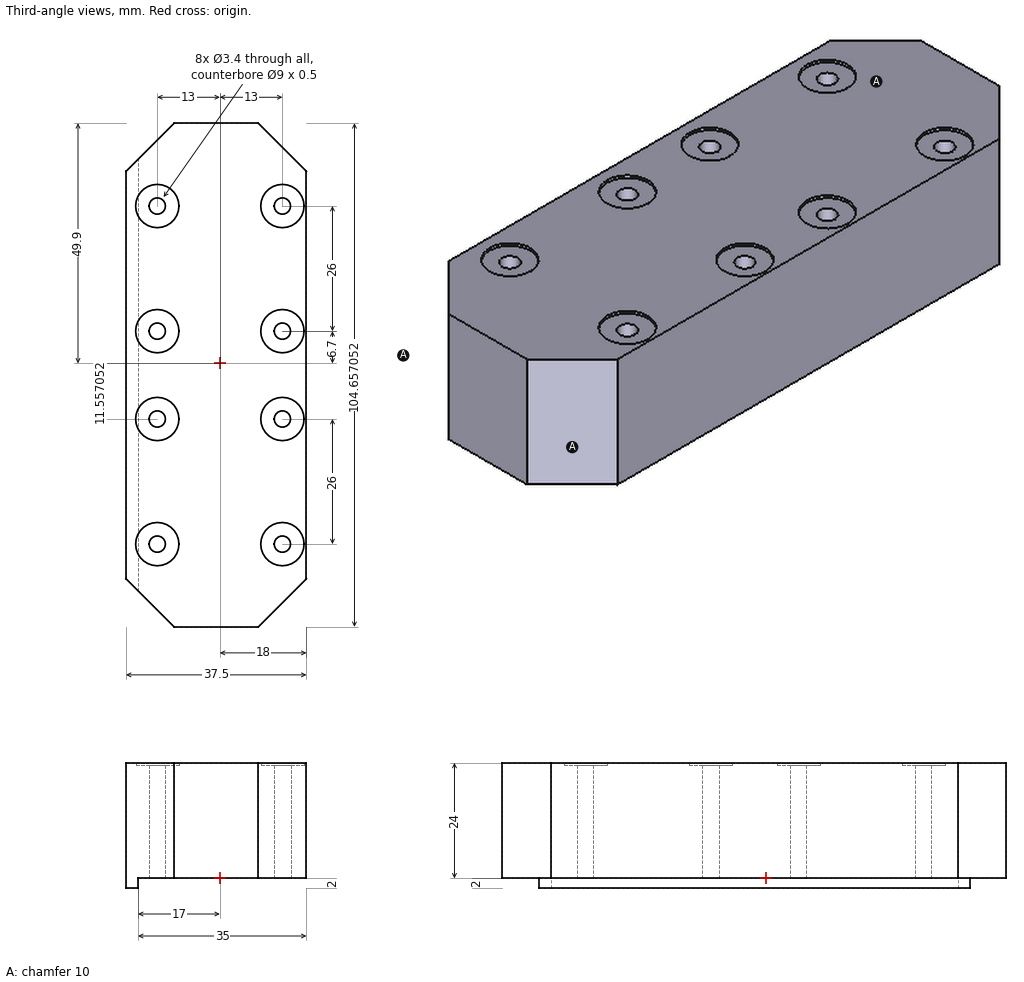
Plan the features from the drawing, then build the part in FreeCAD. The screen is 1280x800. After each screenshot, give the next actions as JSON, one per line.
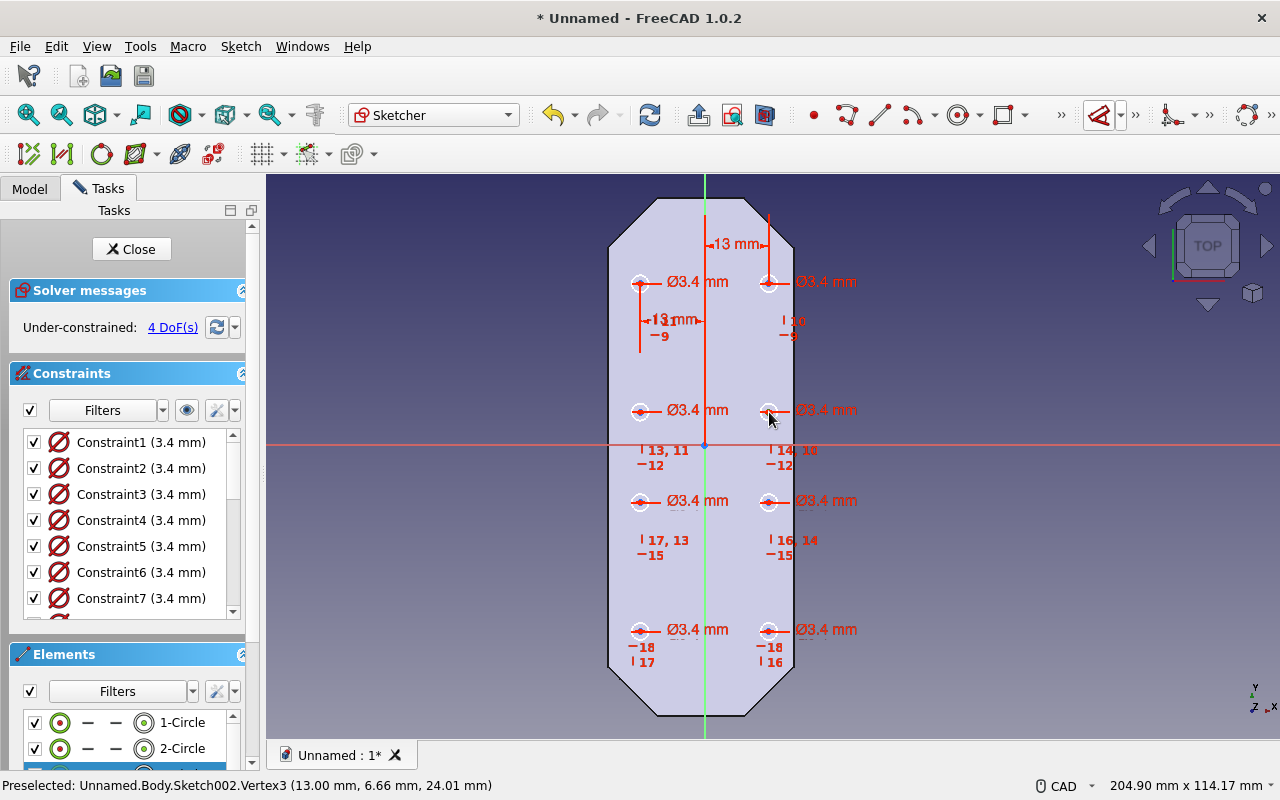
{"action": "left_click", "coordinate": [1120, 116]}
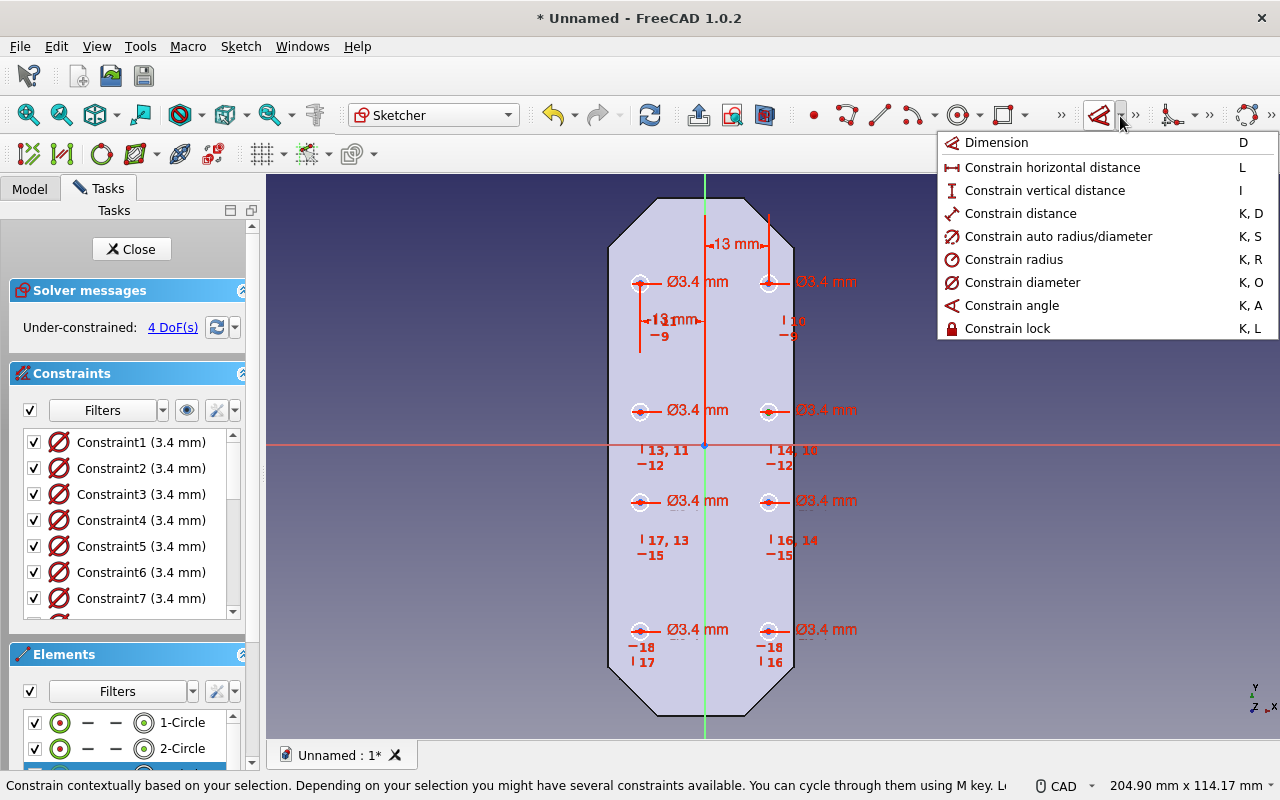
{"action": "left_click", "coordinate": [1108, 190]}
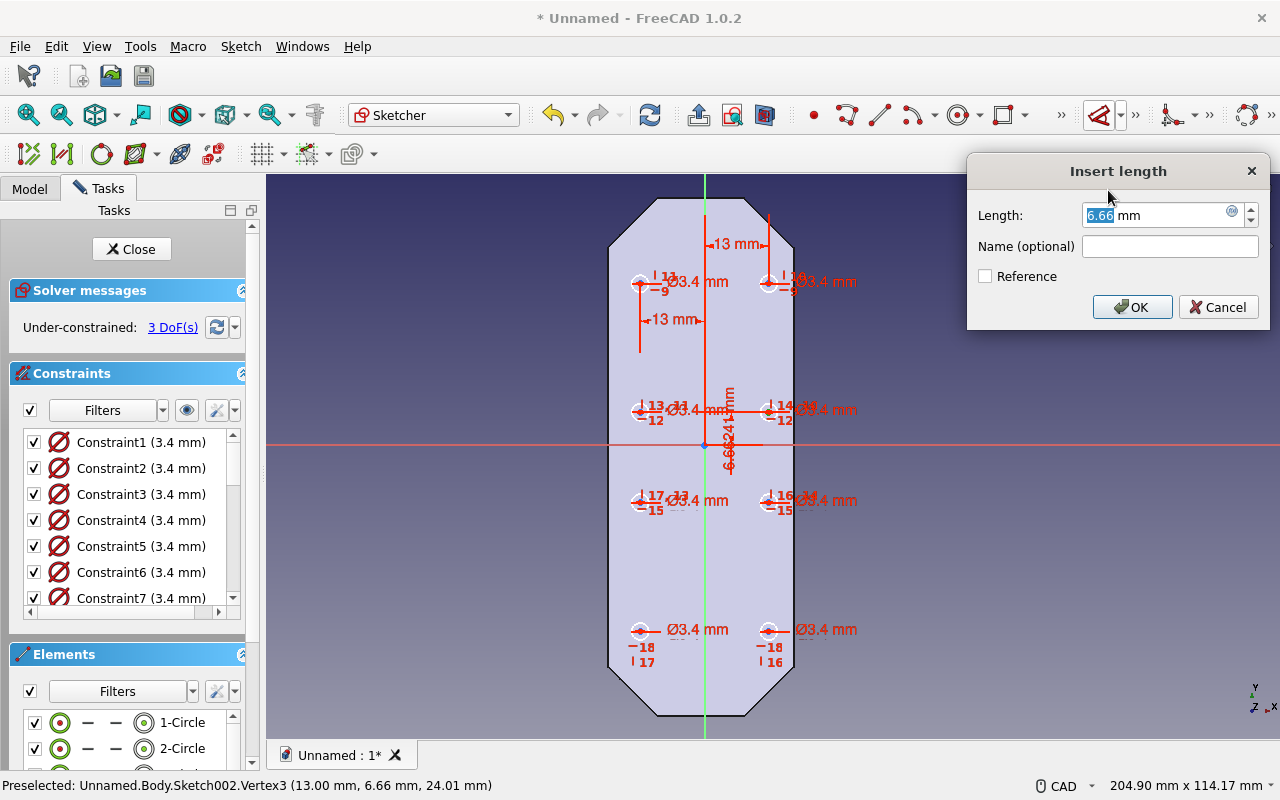
{"action": "type", "text": "6.7"}
{"action": "key", "text": "Return"}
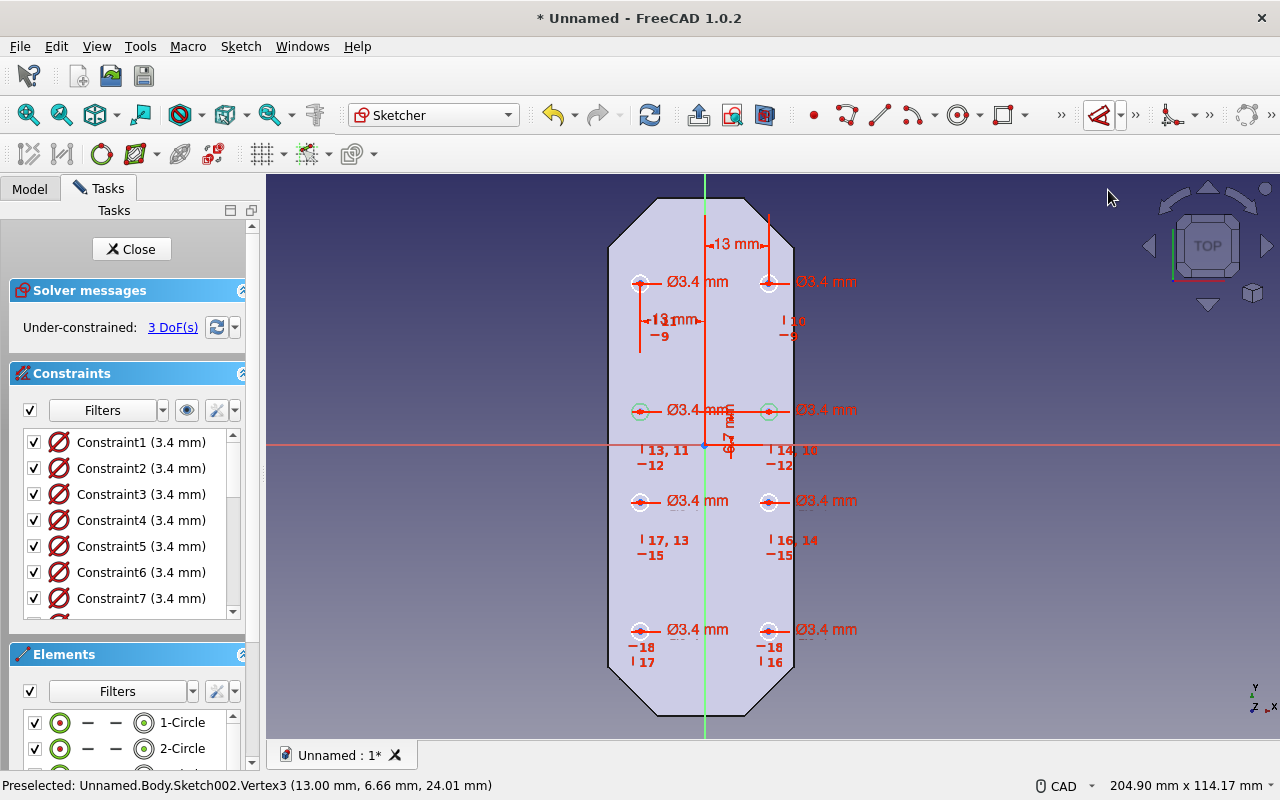
{"action": "left_click", "coordinate": [769, 284]}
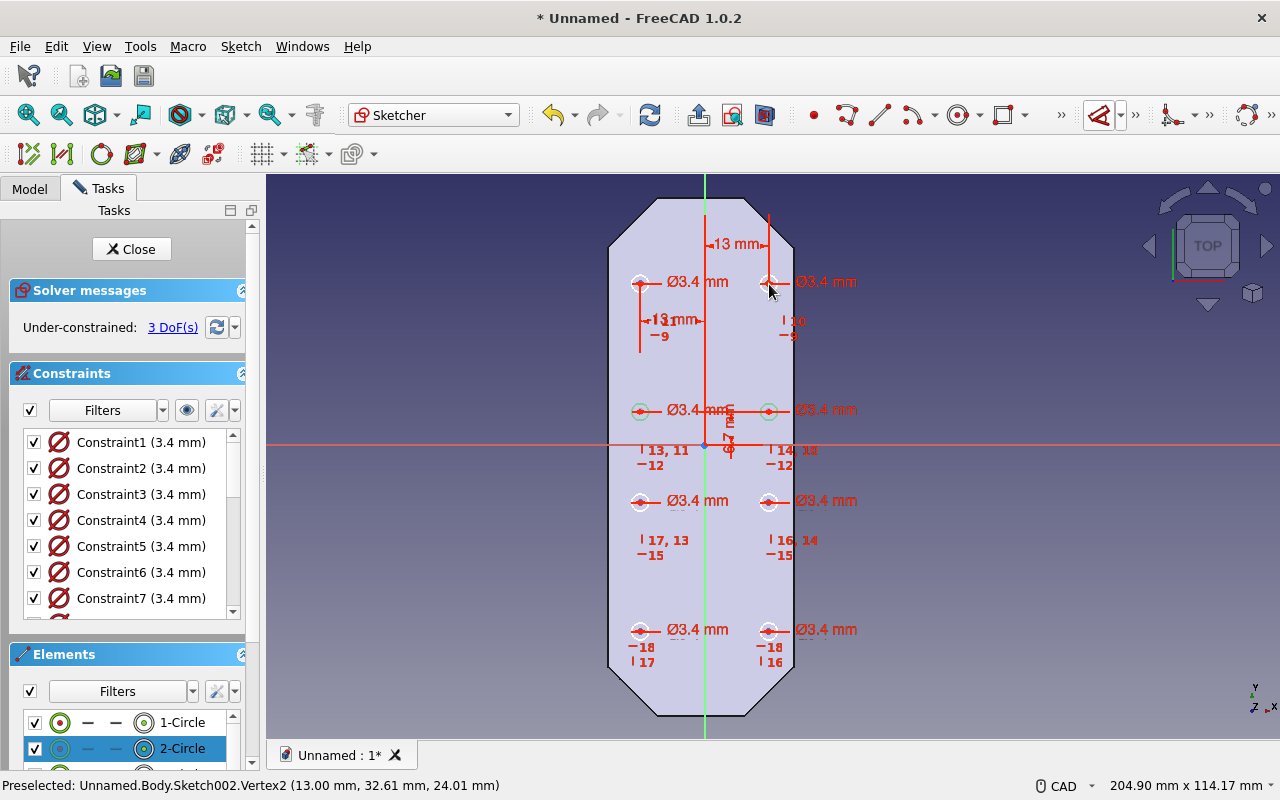
{"action": "left_click", "coordinate": [769, 412]}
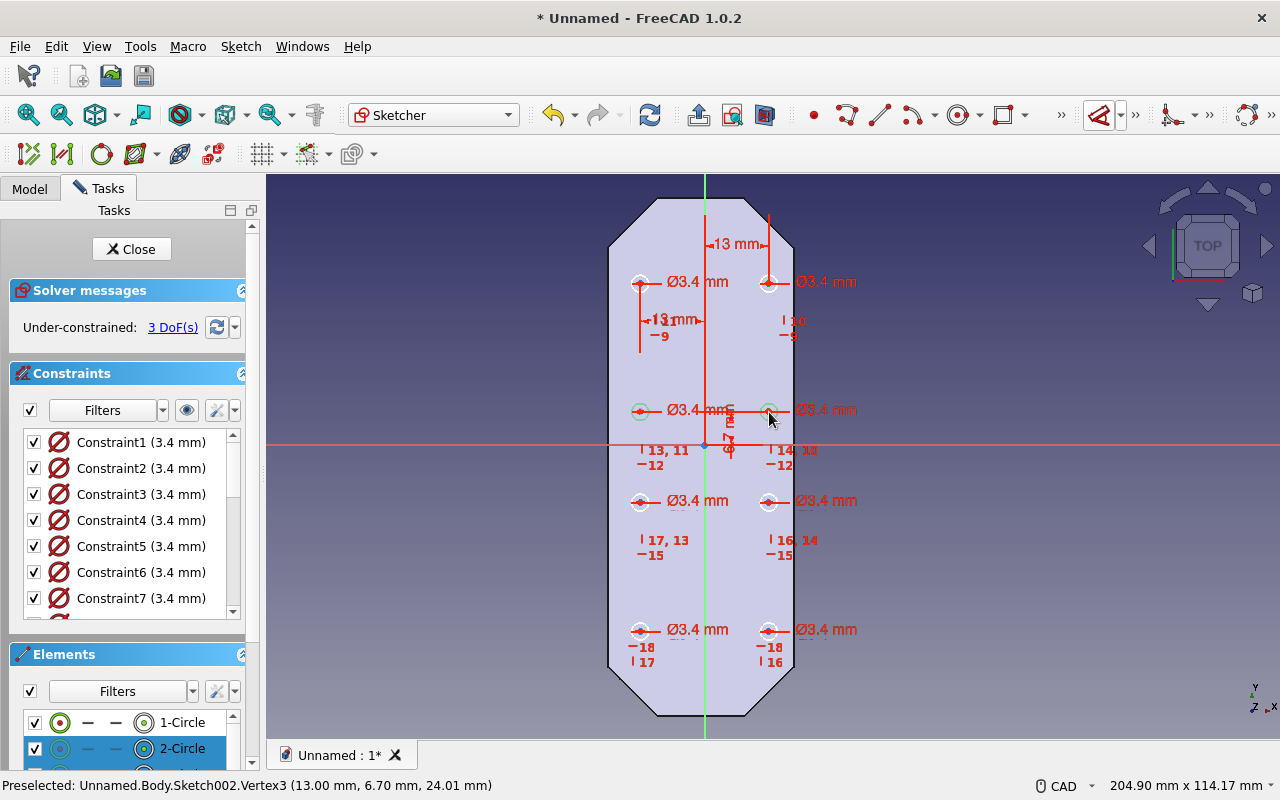
{"action": "key", "text": "i"}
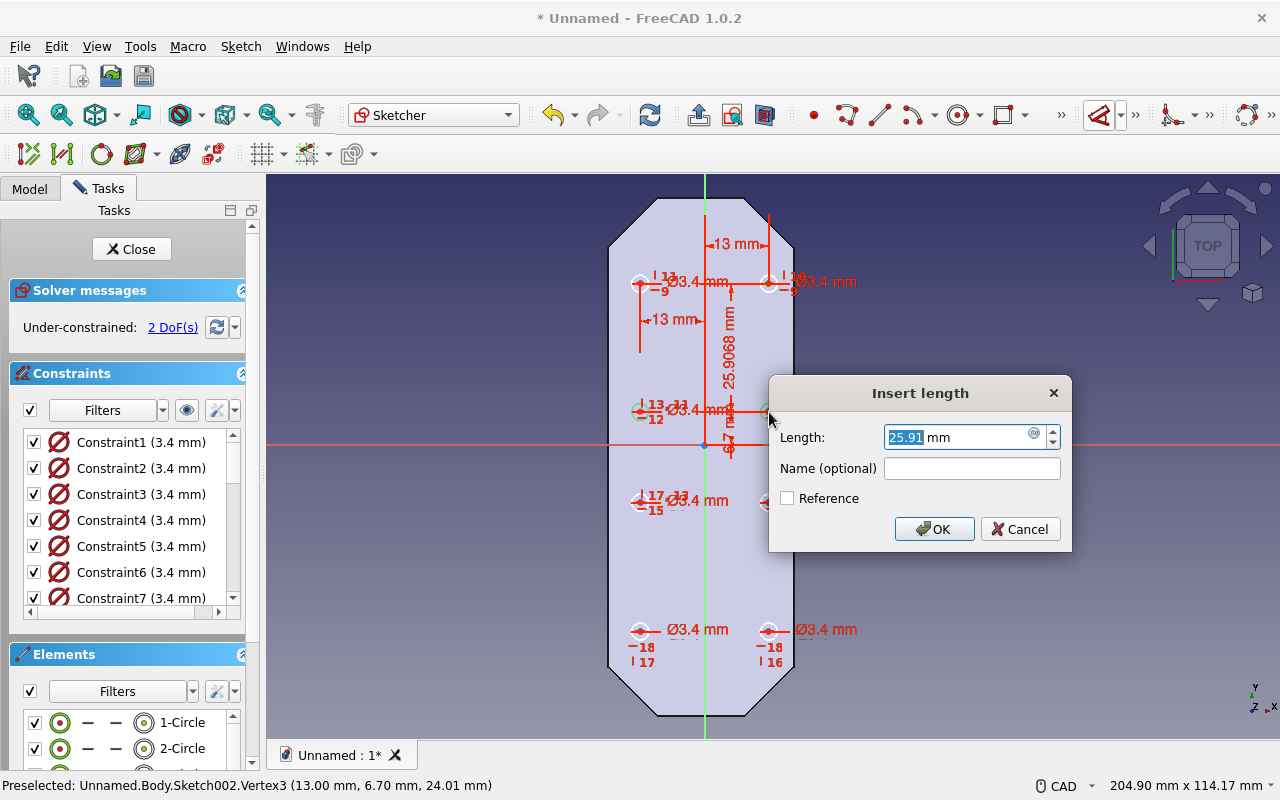
{"action": "type", "text": "26"}
{"action": "key", "text": "Return"}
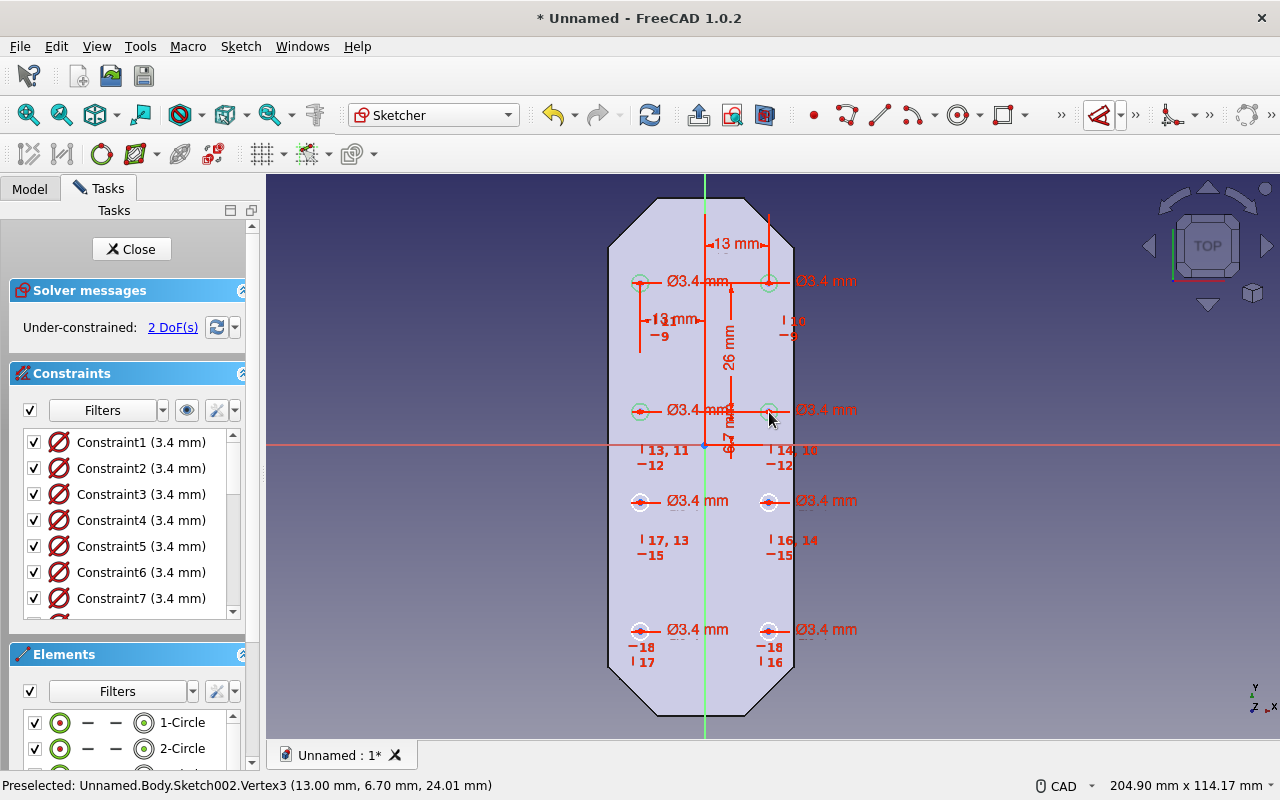
{"action": "left_click", "coordinate": [769, 503]}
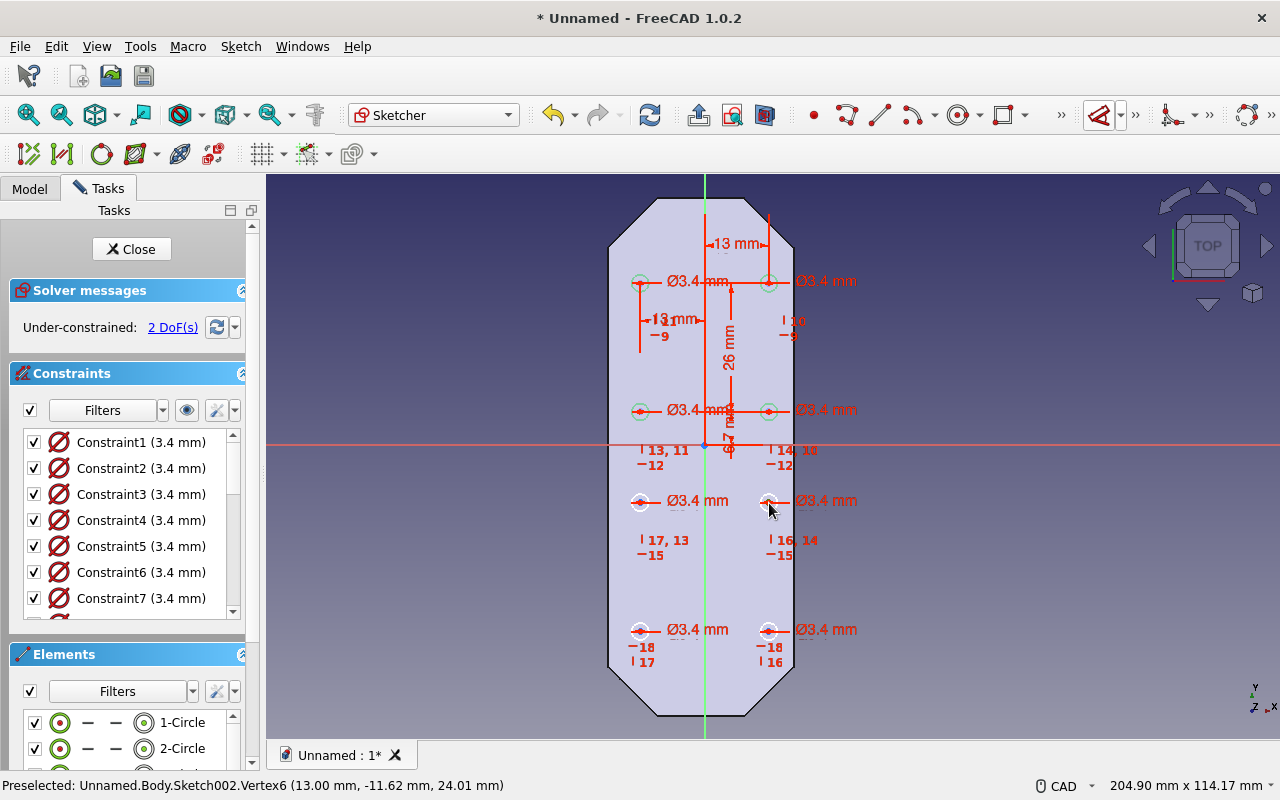
{"action": "left_click", "coordinate": [769, 632]}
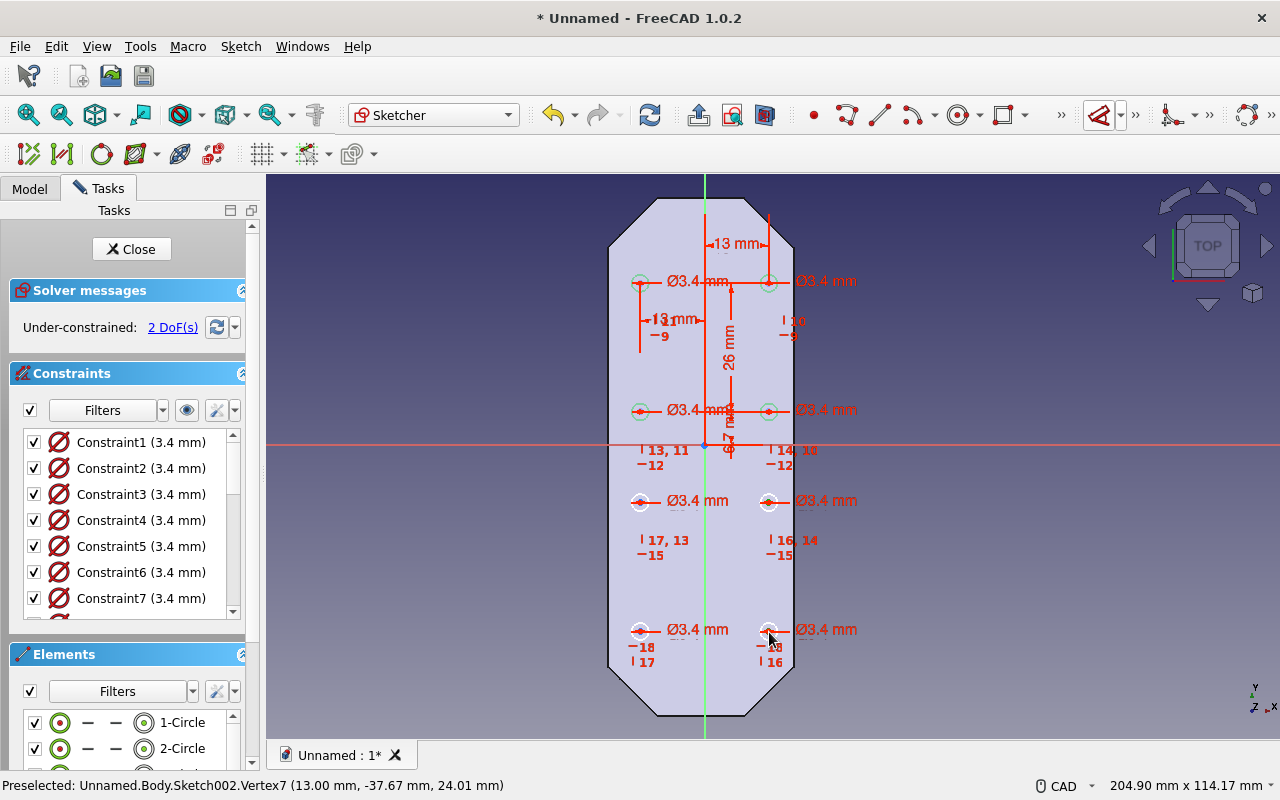
{"action": "key", "text": "i"}